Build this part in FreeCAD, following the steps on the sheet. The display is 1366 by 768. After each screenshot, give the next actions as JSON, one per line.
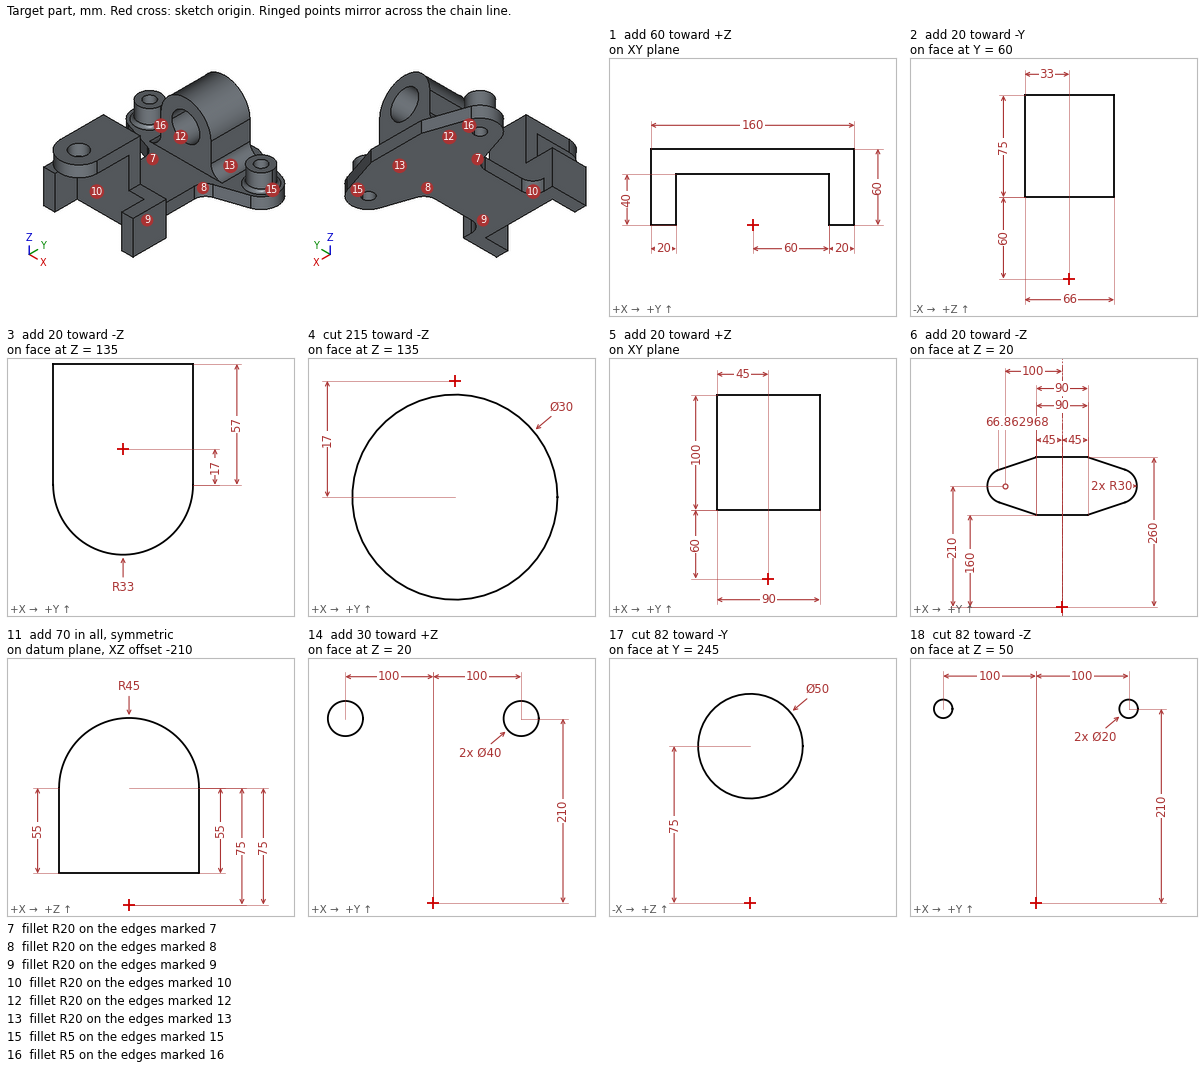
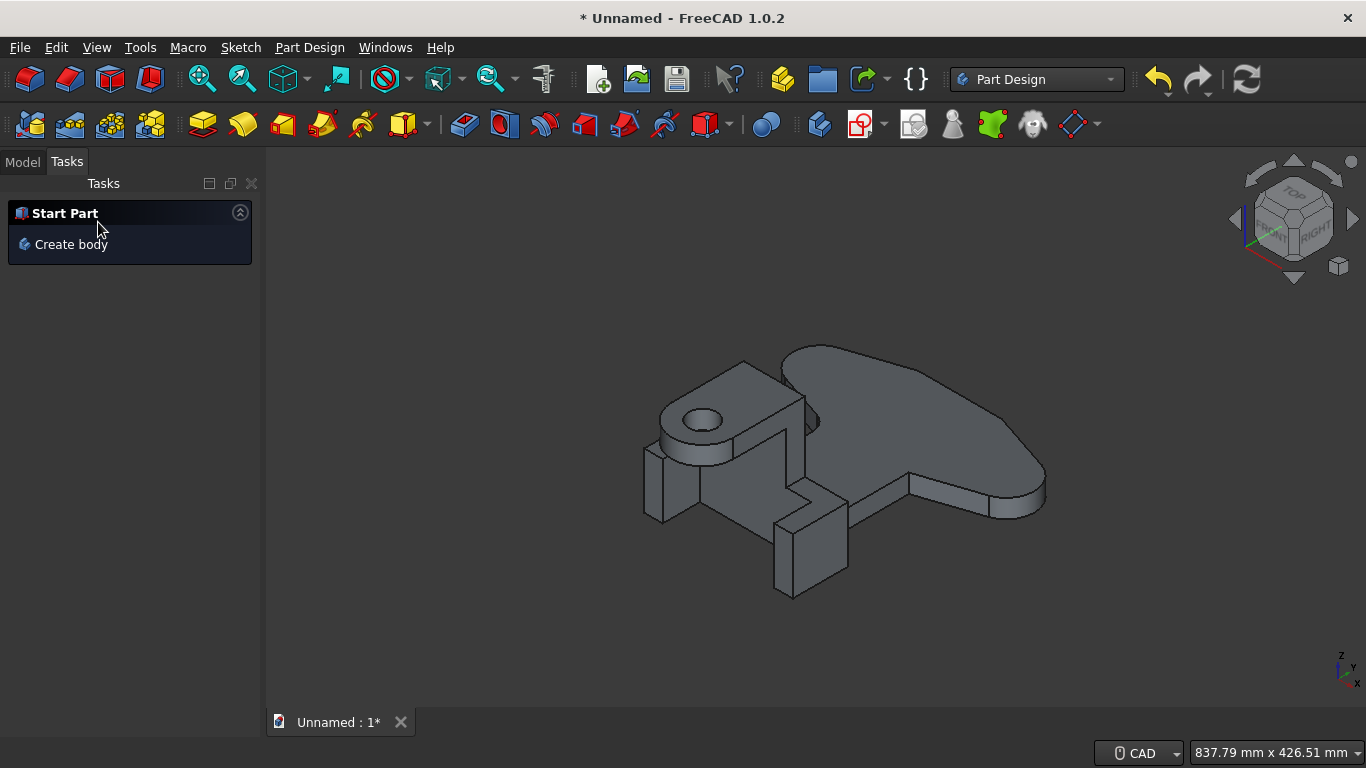
{"action": "key", "text": "2"}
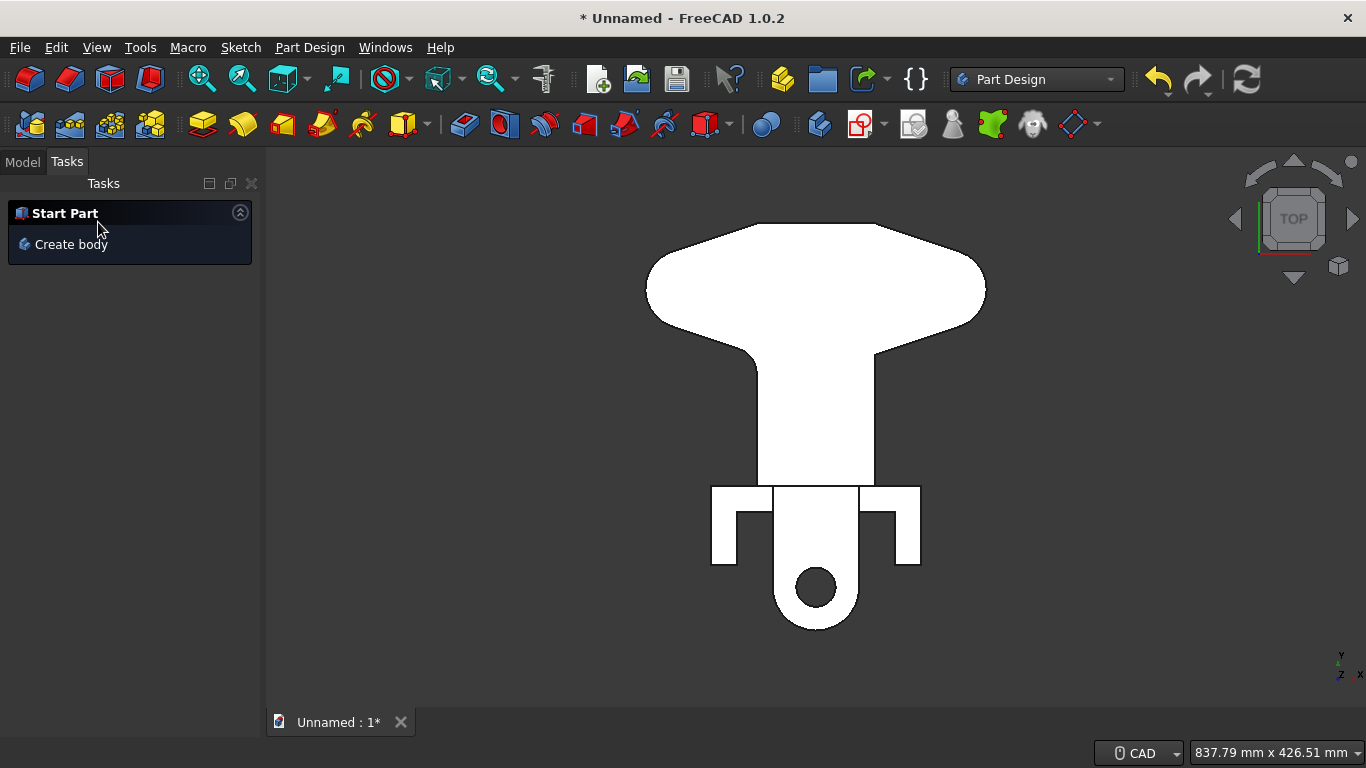
{"action": "key", "text": "0"}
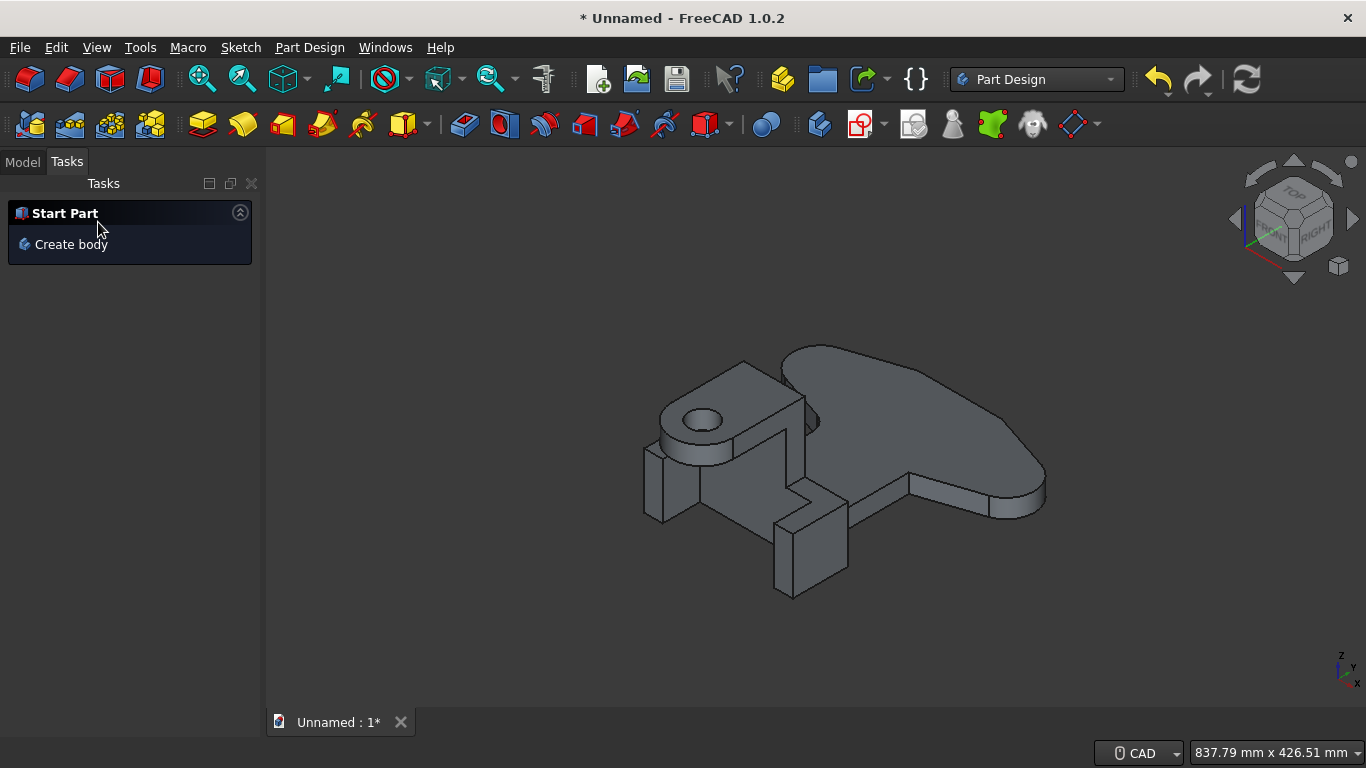
{"action": "key", "text": "1"}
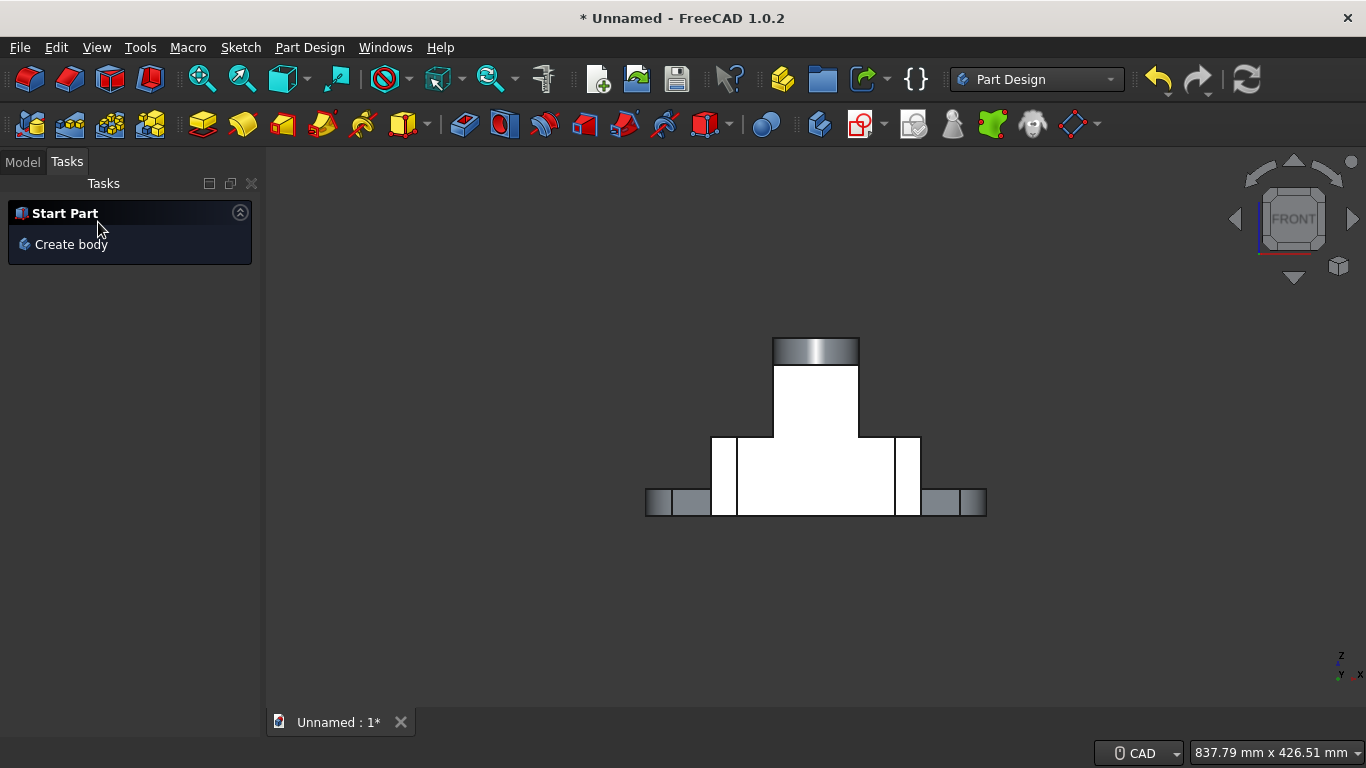
{"action": "key", "text": "v f"}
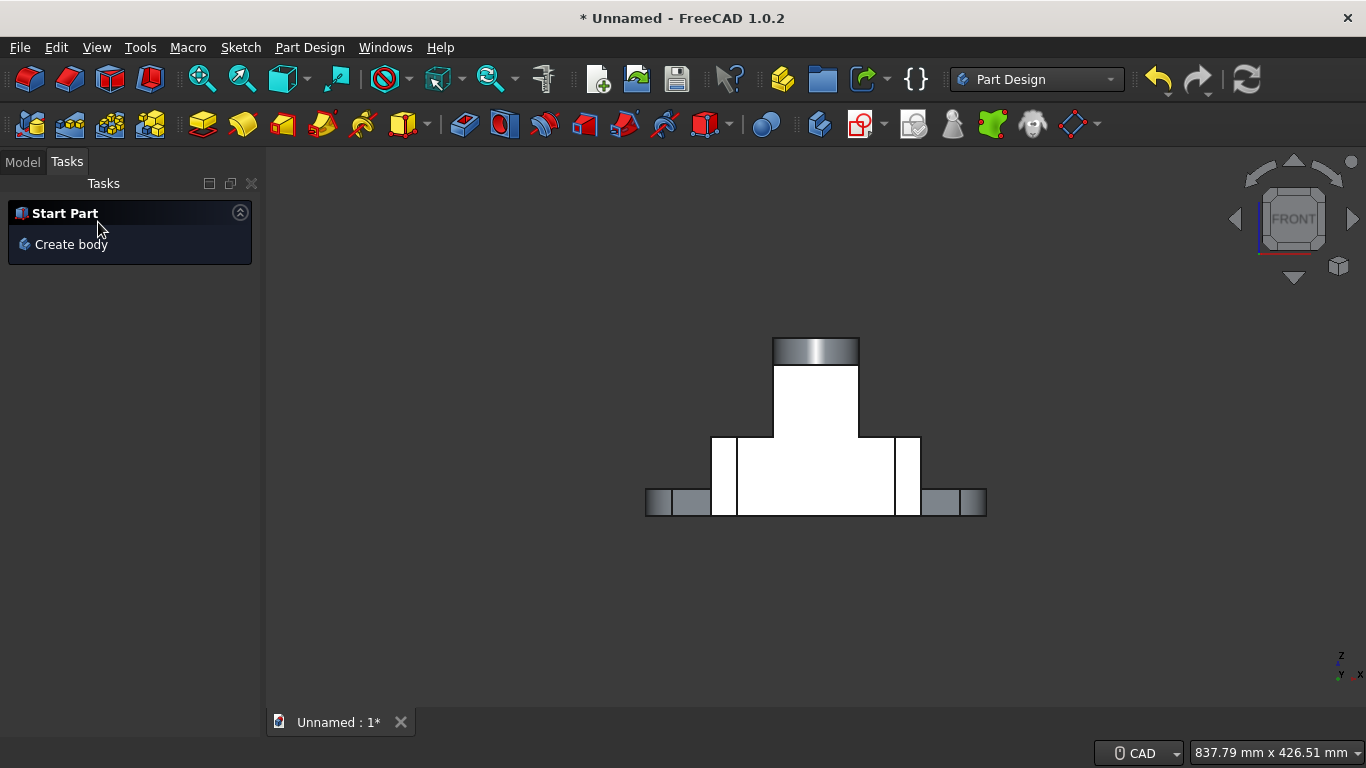
{"action": "key", "text": "3"}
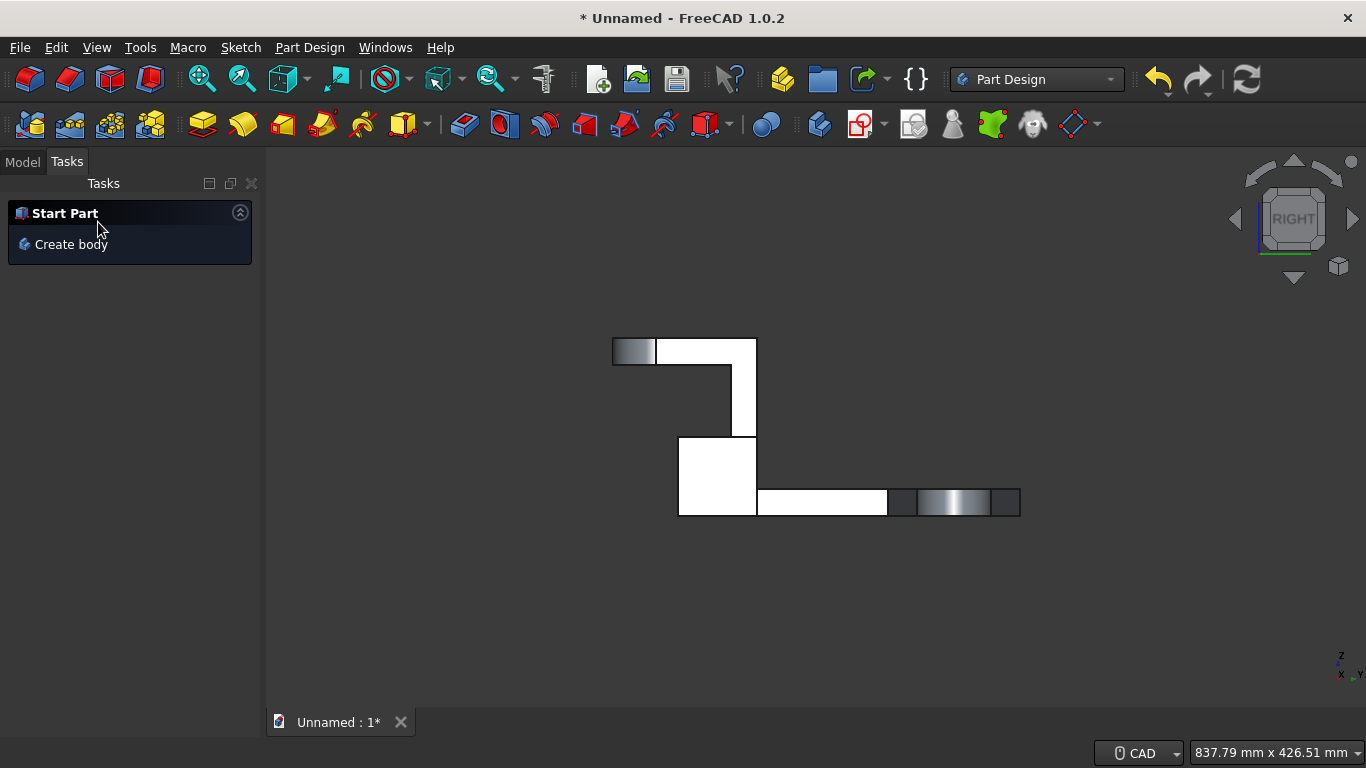
{"action": "key", "text": "v f"}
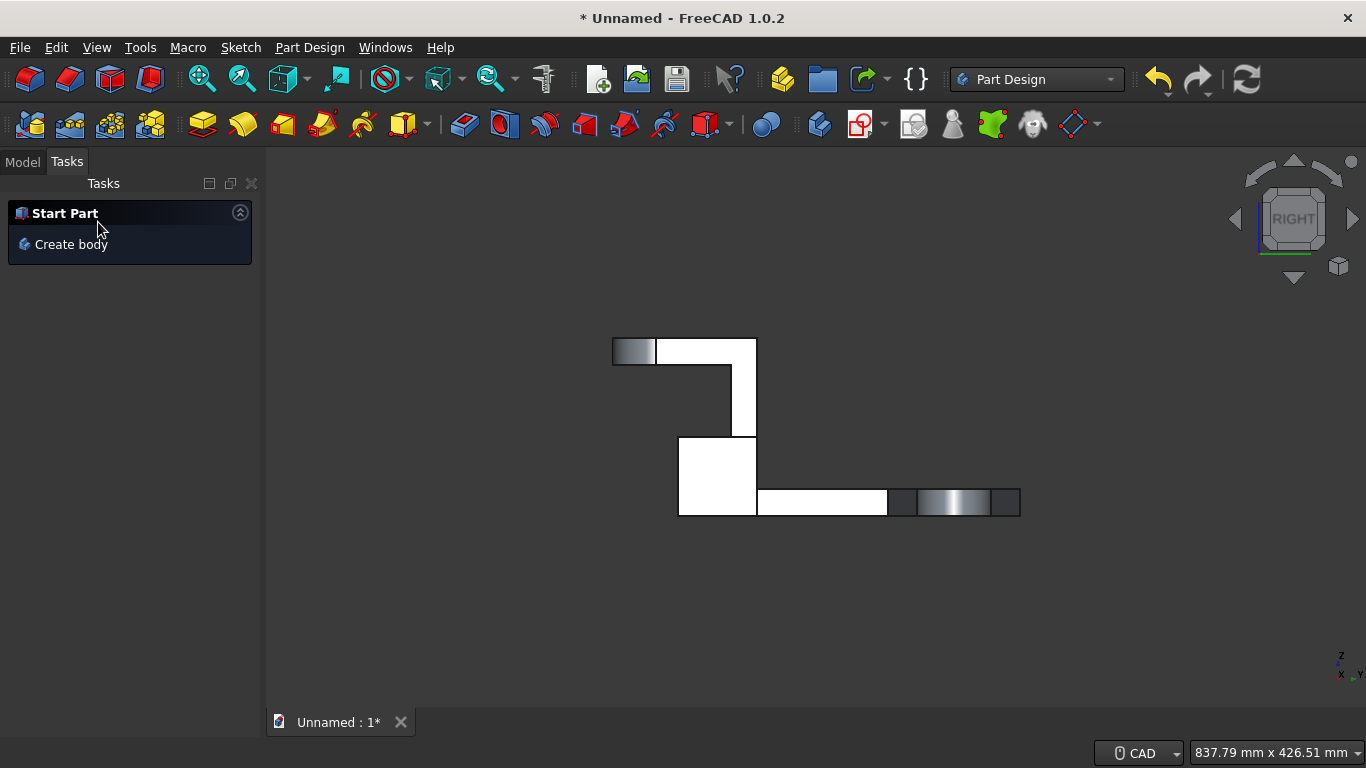
{"action": "key", "text": "5"}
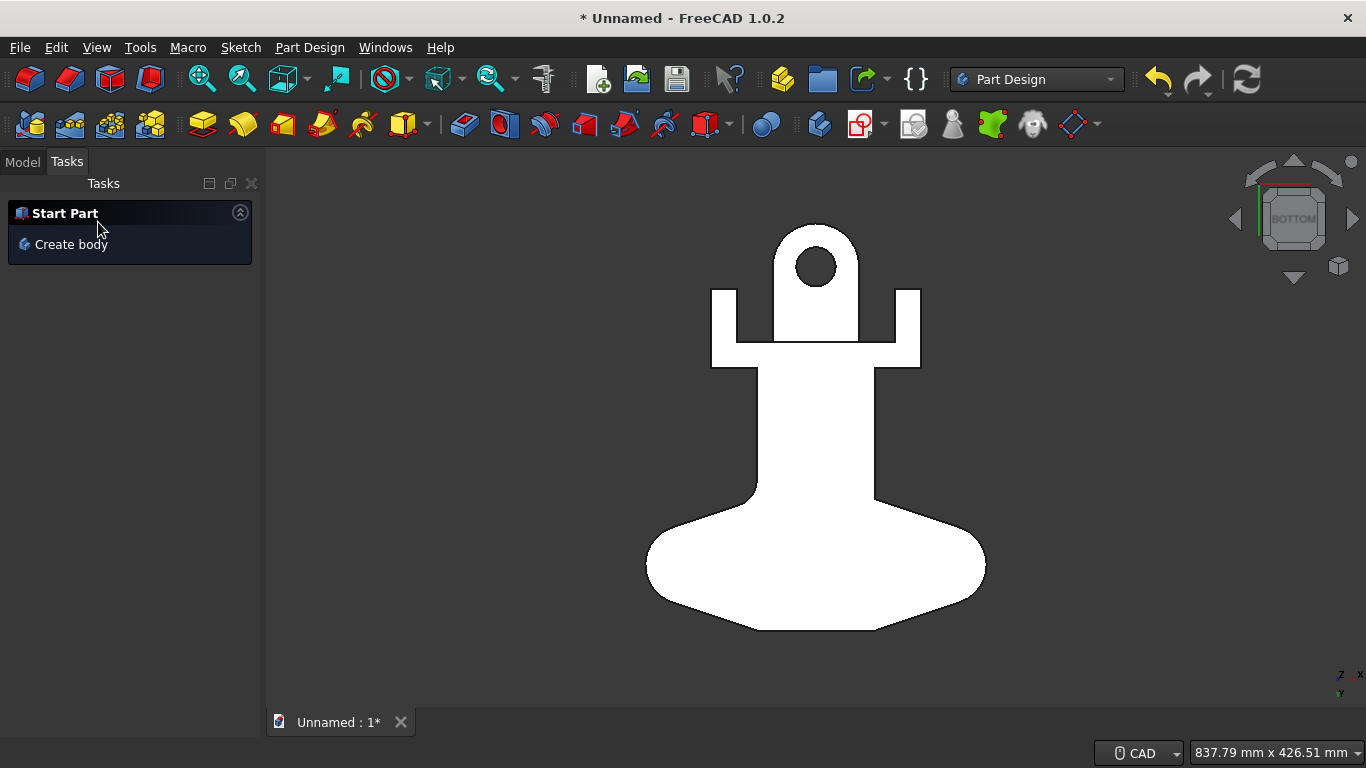
{"action": "key", "text": "4"}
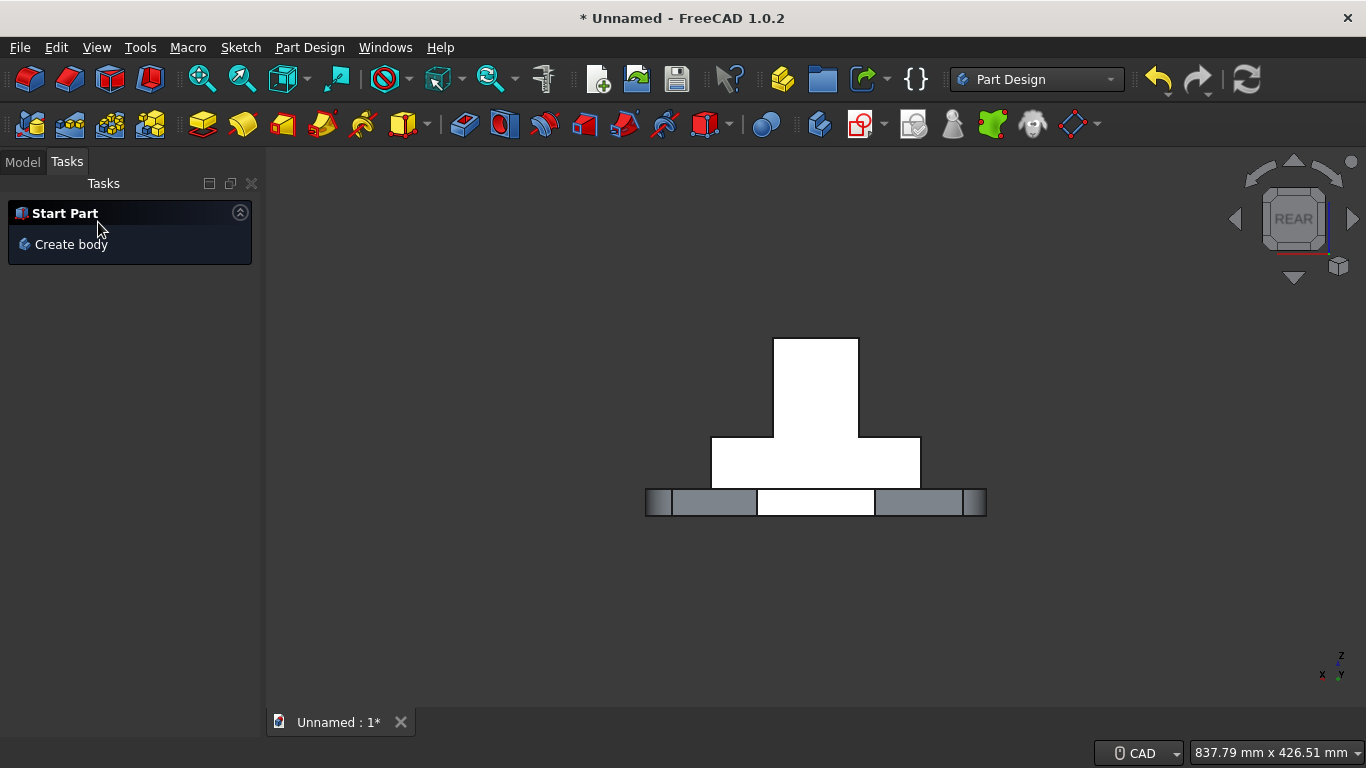
{"action": "key", "text": "v f"}